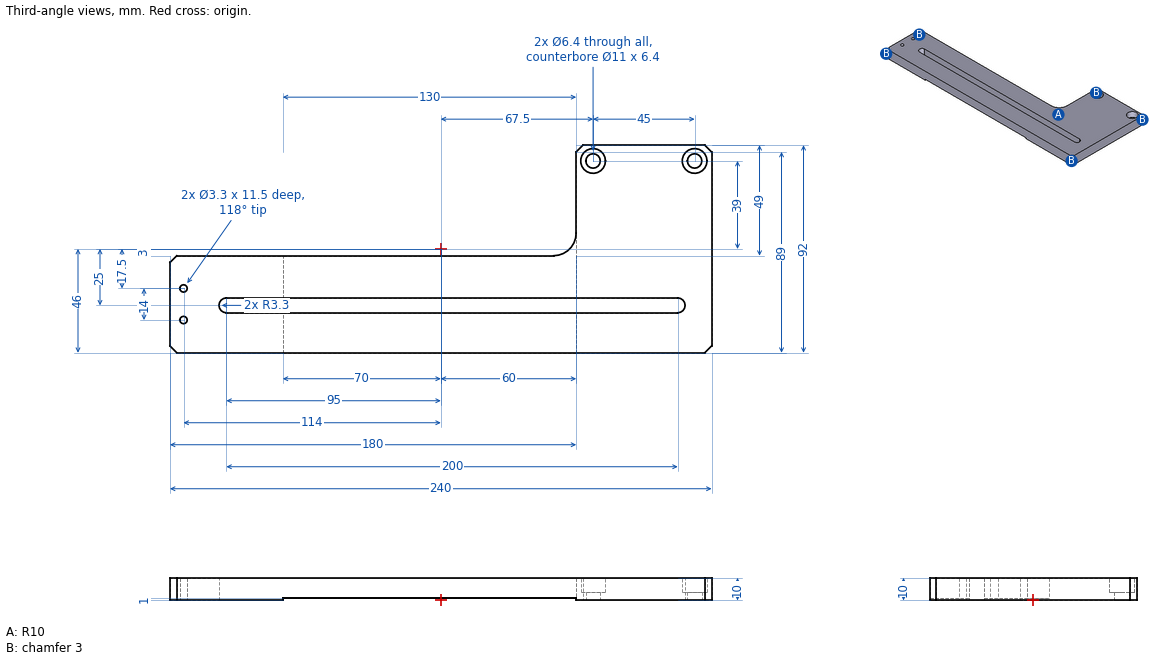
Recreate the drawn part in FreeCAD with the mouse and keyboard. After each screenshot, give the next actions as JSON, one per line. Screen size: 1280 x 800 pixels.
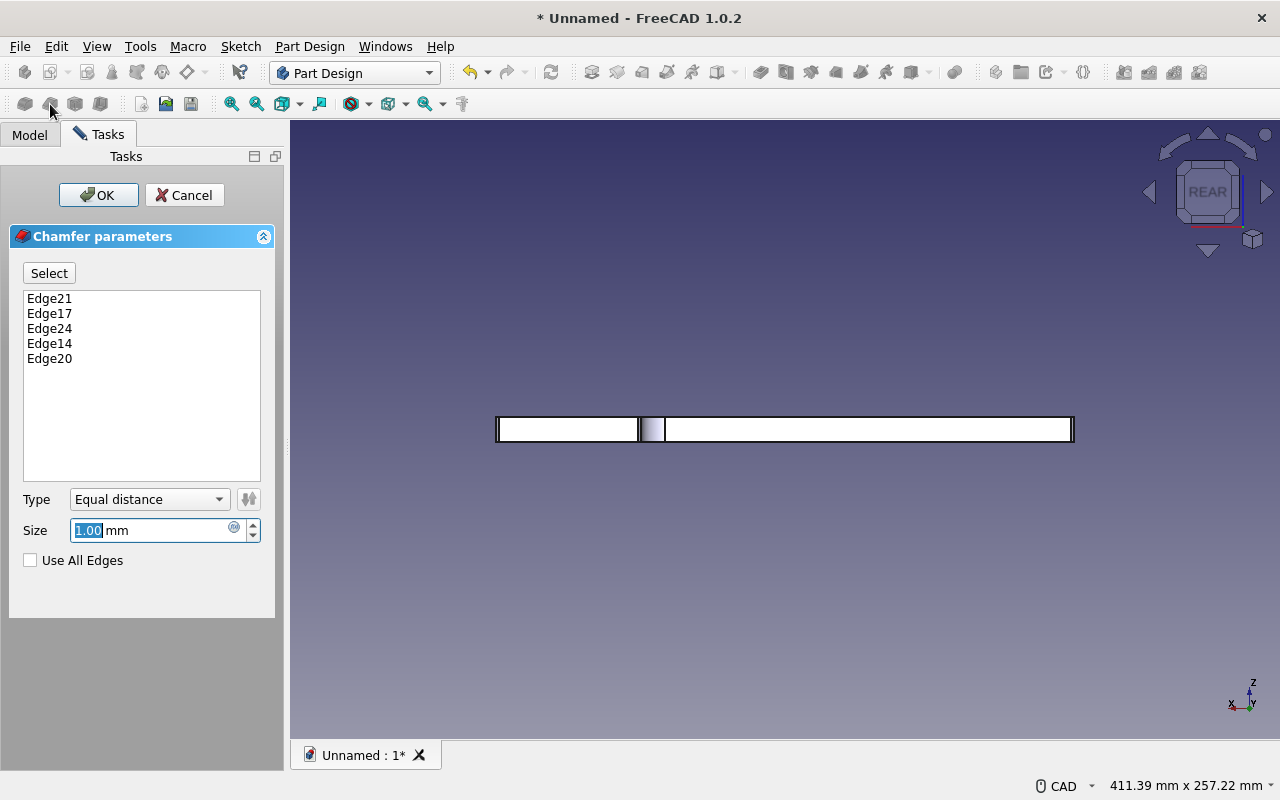
{"action": "type", "text": "3"}
{"action": "key", "text": "Tab"}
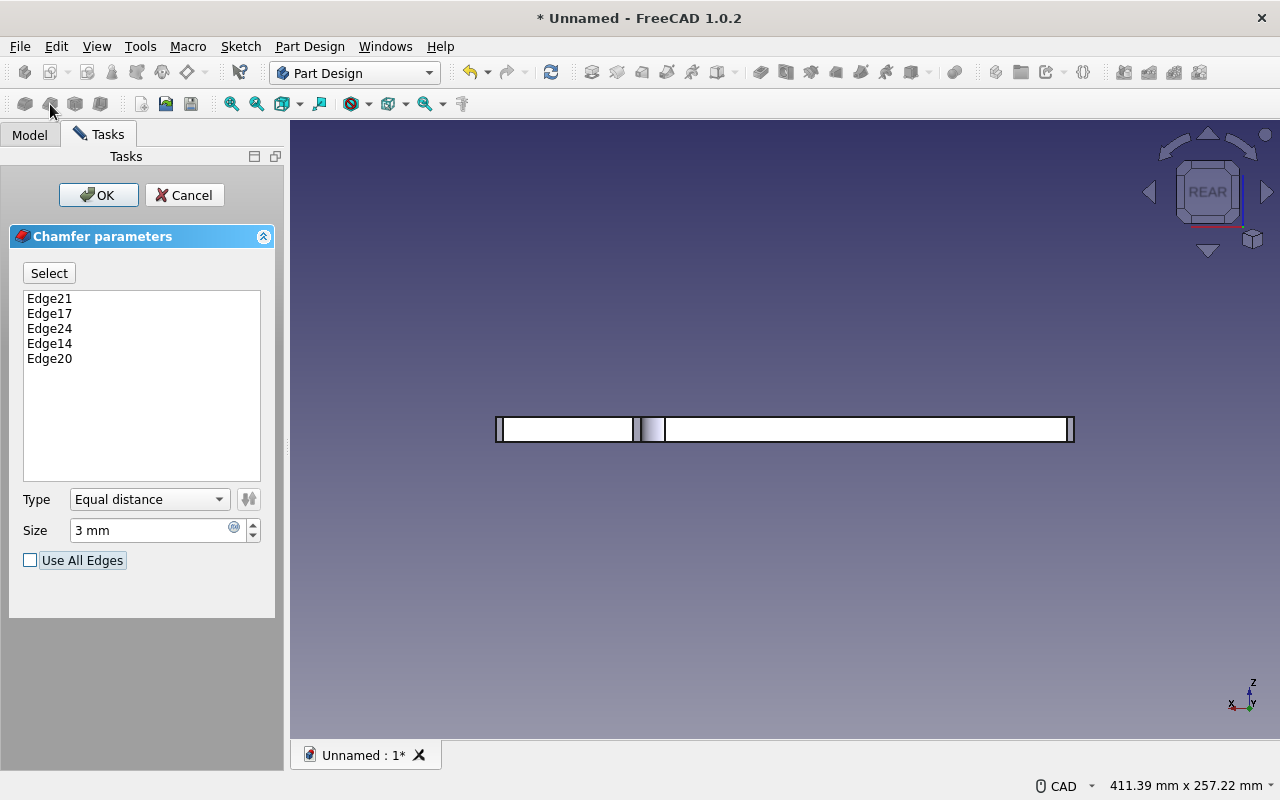
{"action": "left_click", "coordinate": [99, 195]}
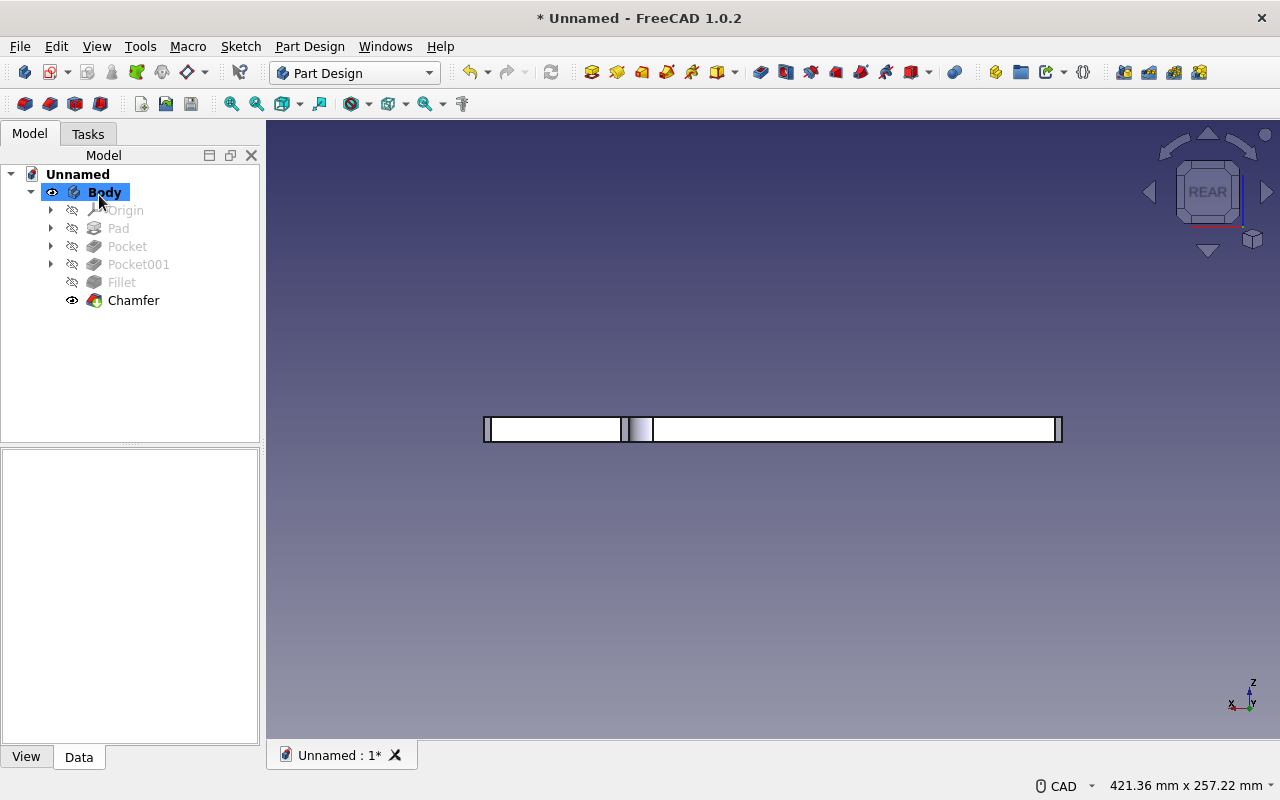
{"action": "key", "text": "0"}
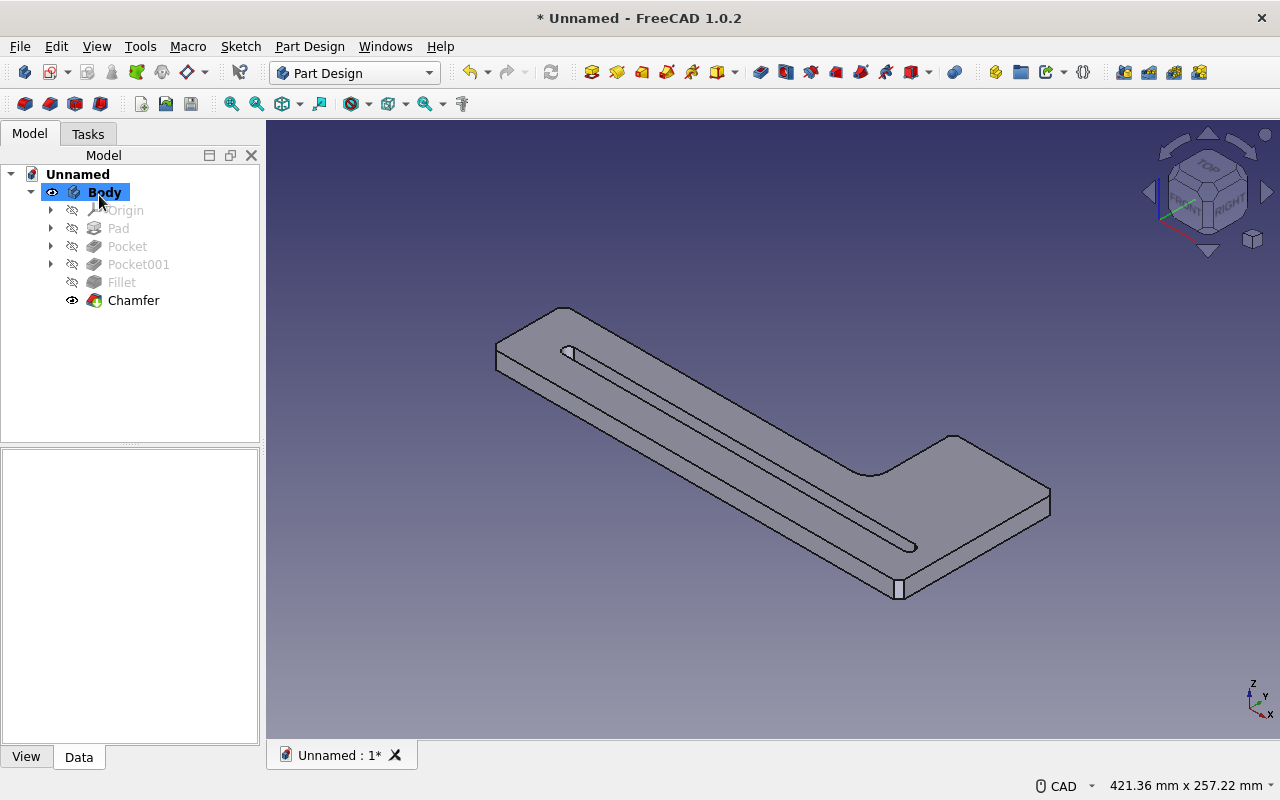
{"action": "left_click", "coordinate": [993, 494]}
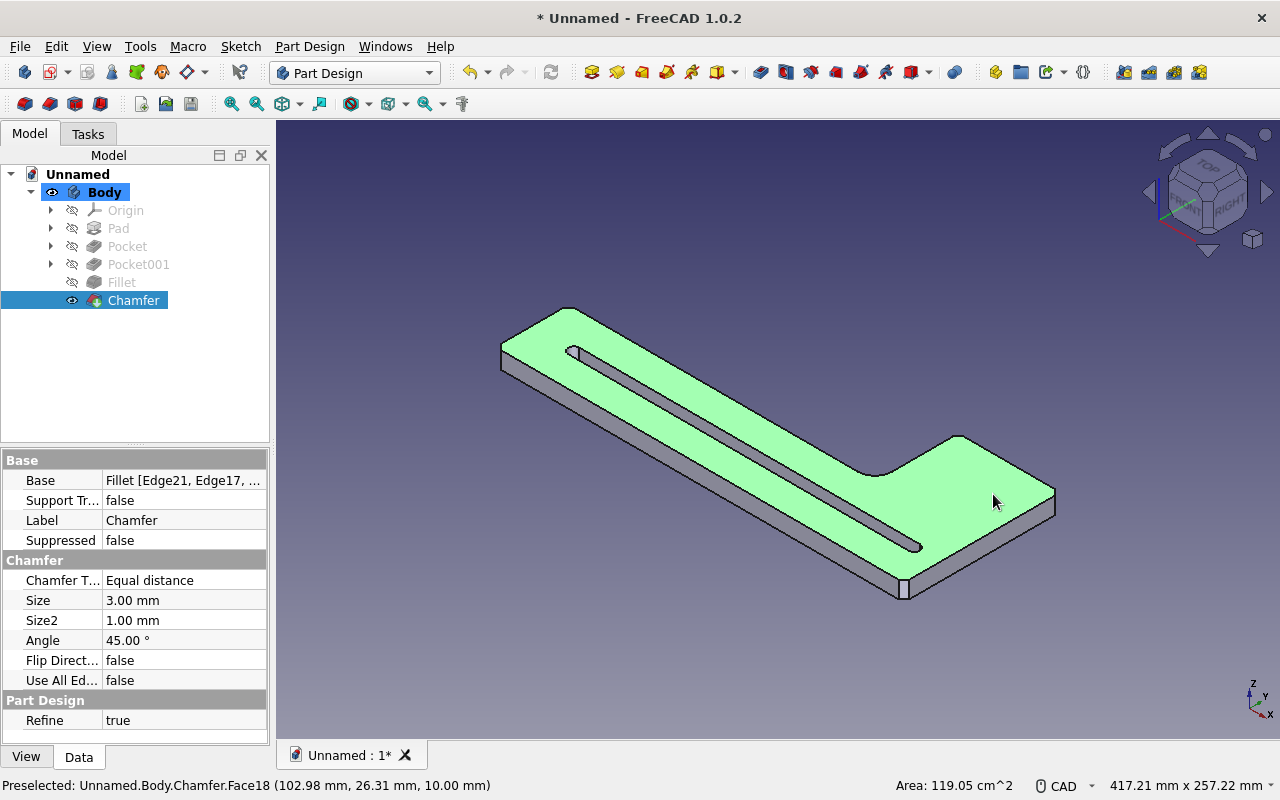
{"action": "left_click", "coordinate": [50, 72]}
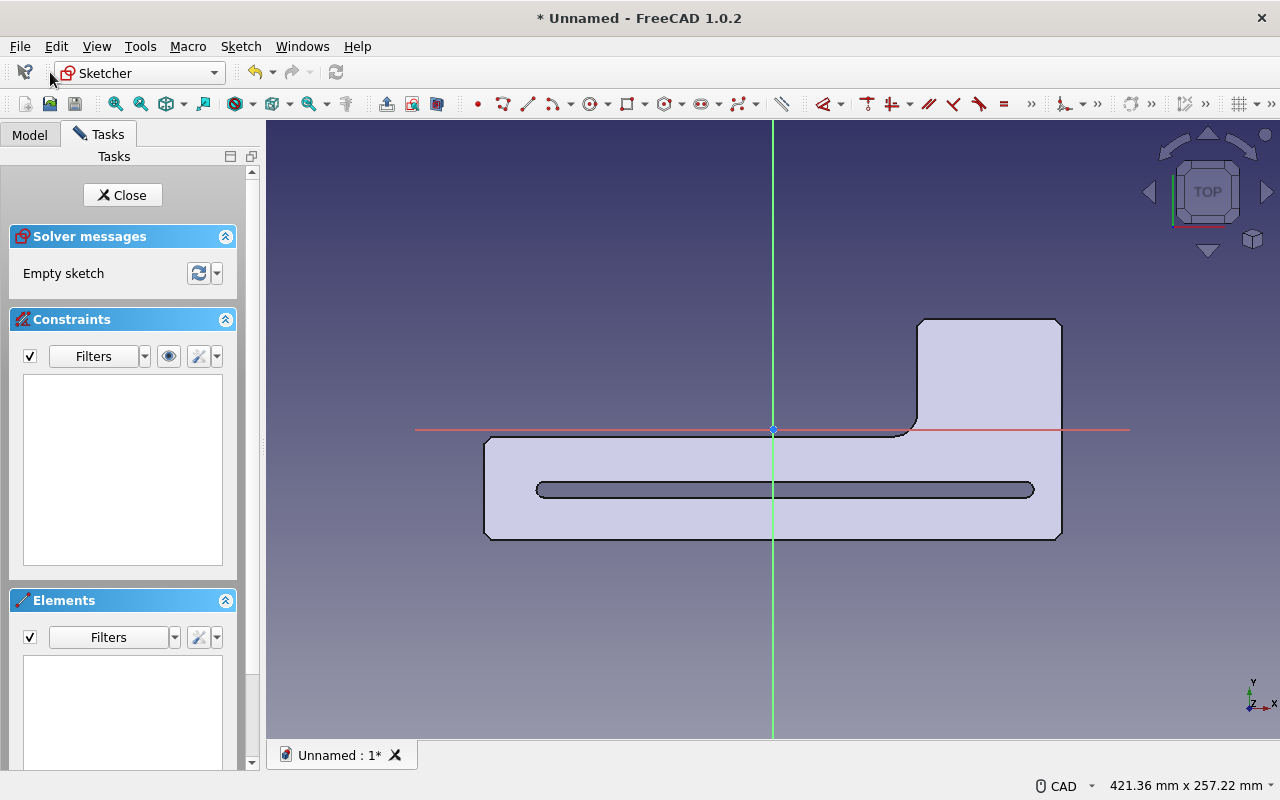
{"action": "scroll", "coordinate": [473, 496], "scroll_direction": "up", "scroll_amount": 11}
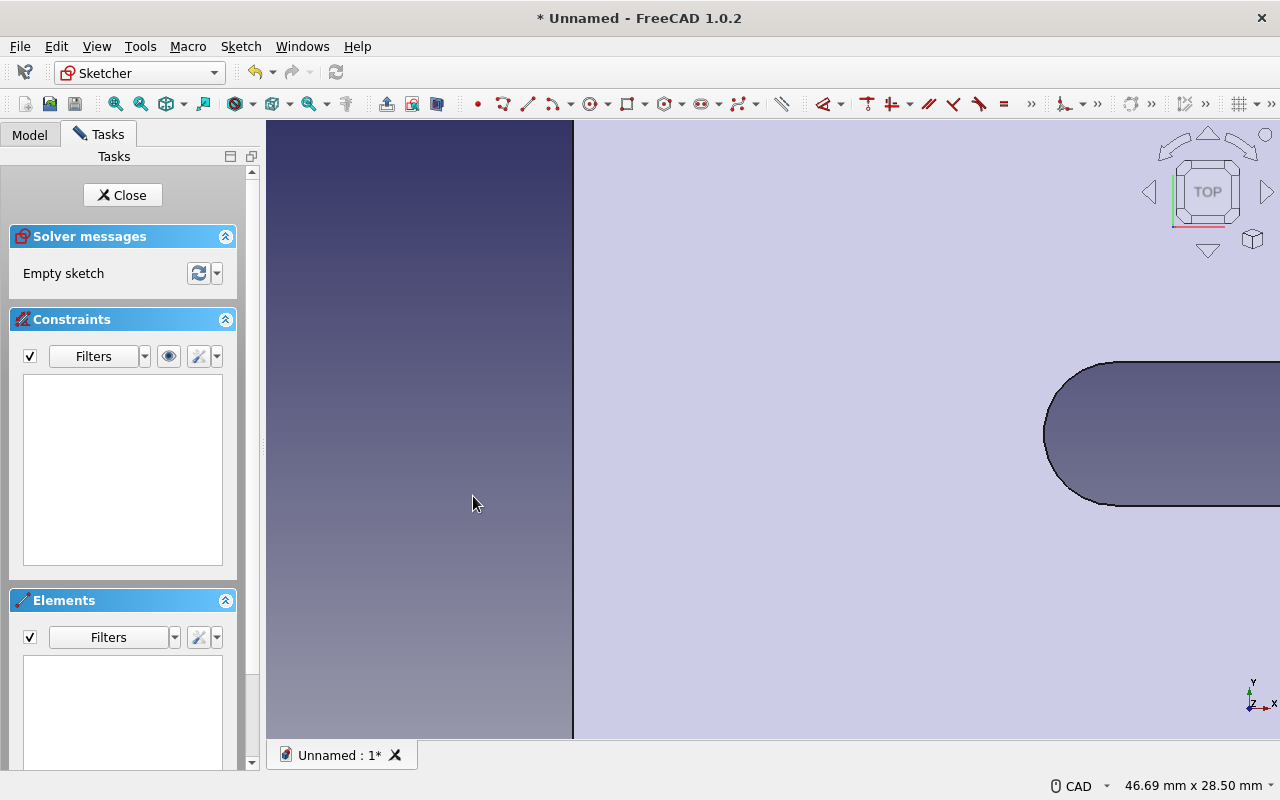
{"action": "left_click", "coordinate": [590, 104]}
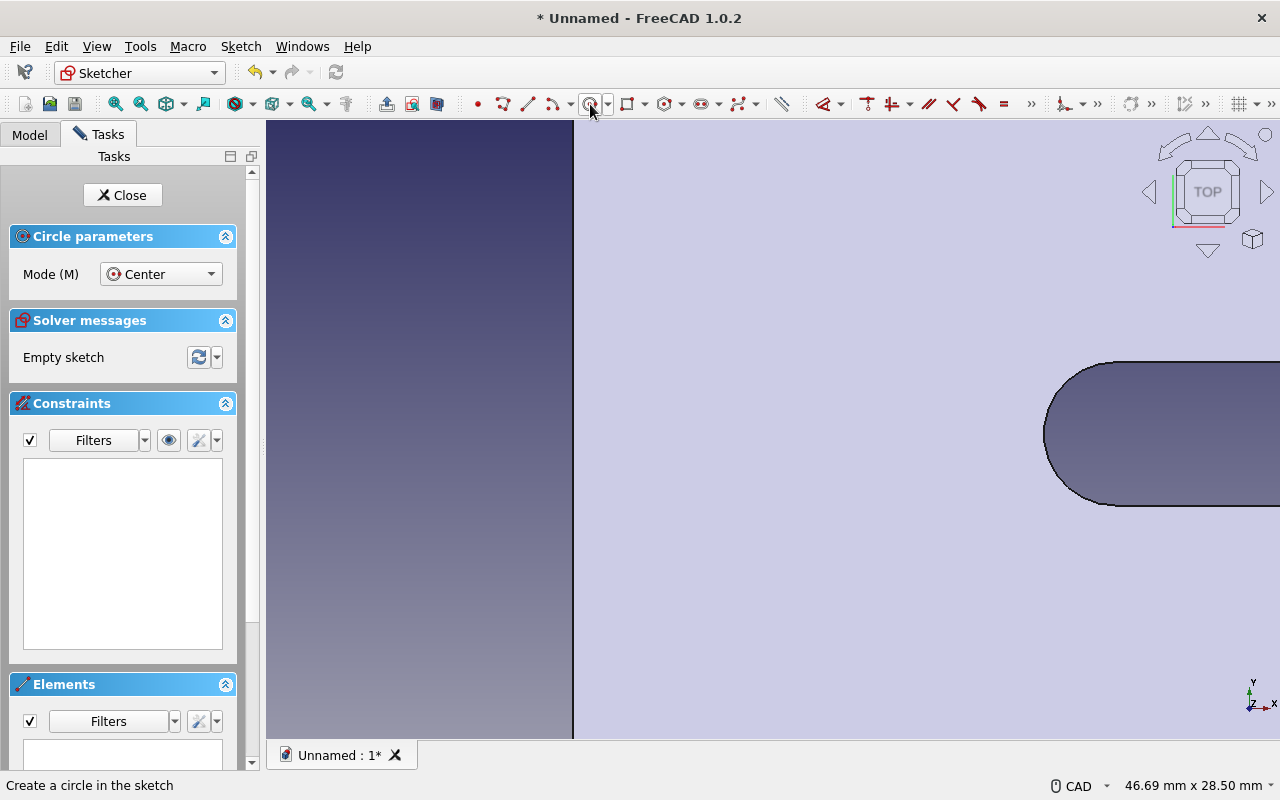
{"action": "left_click", "coordinate": [703, 271]}
{"action": "mouse_move", "coordinate": [728, 246]}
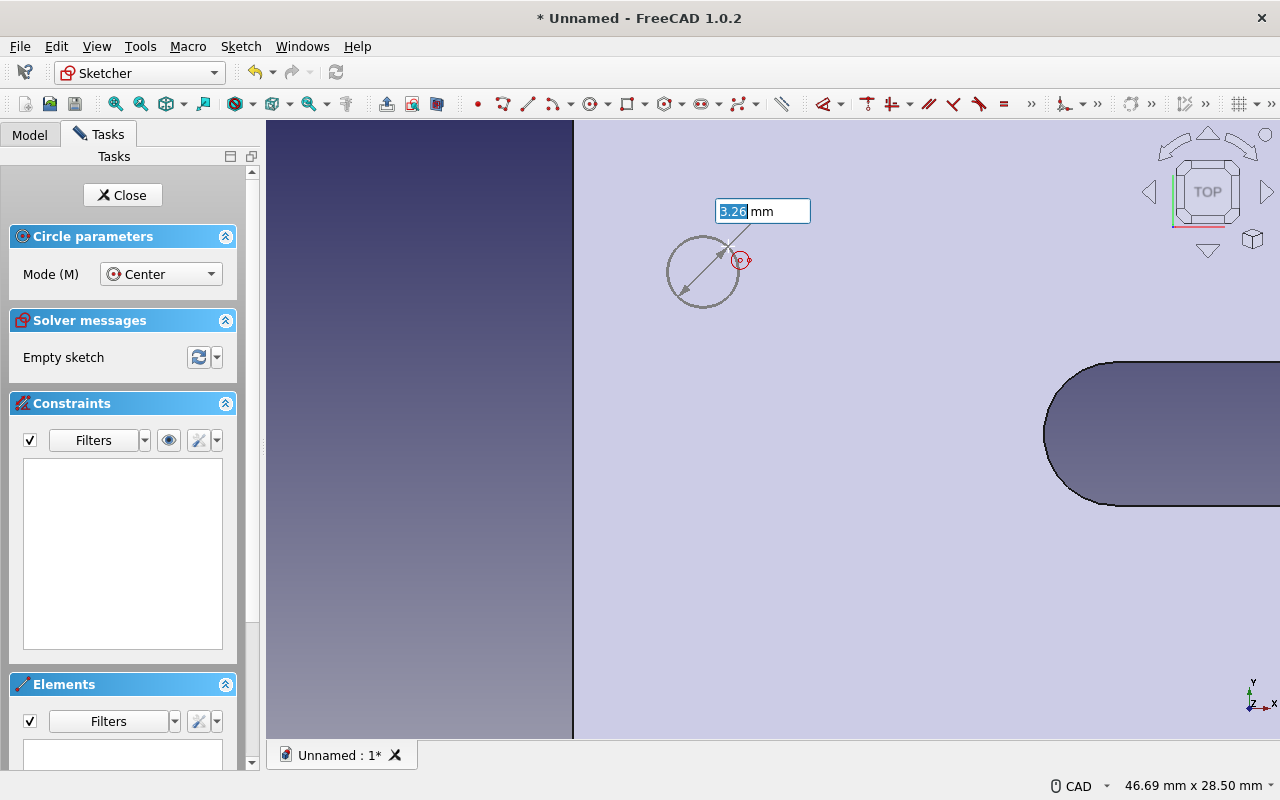
{"action": "type", "text": "3.3"}
{"action": "key", "text": "Return"}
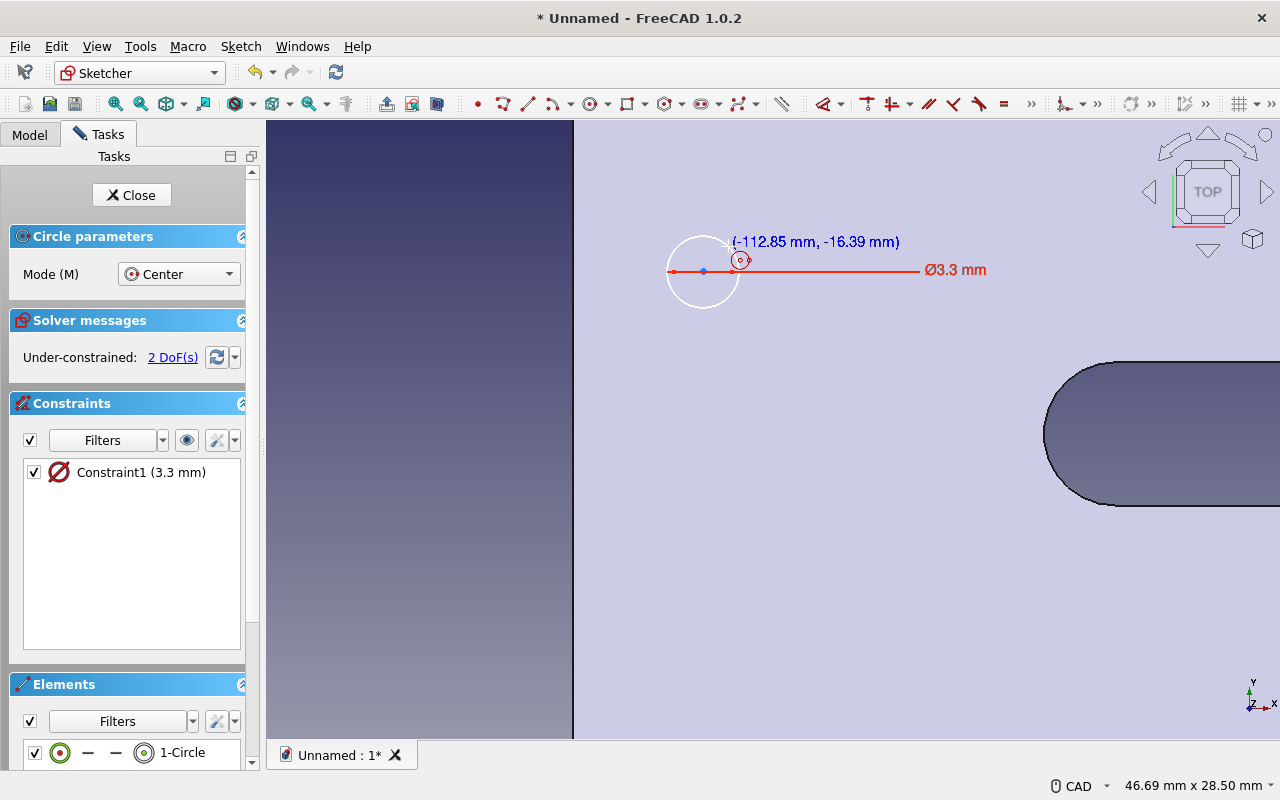
{"action": "left_click", "coordinate": [703, 575]}
{"action": "mouse_move", "coordinate": [728, 550]}